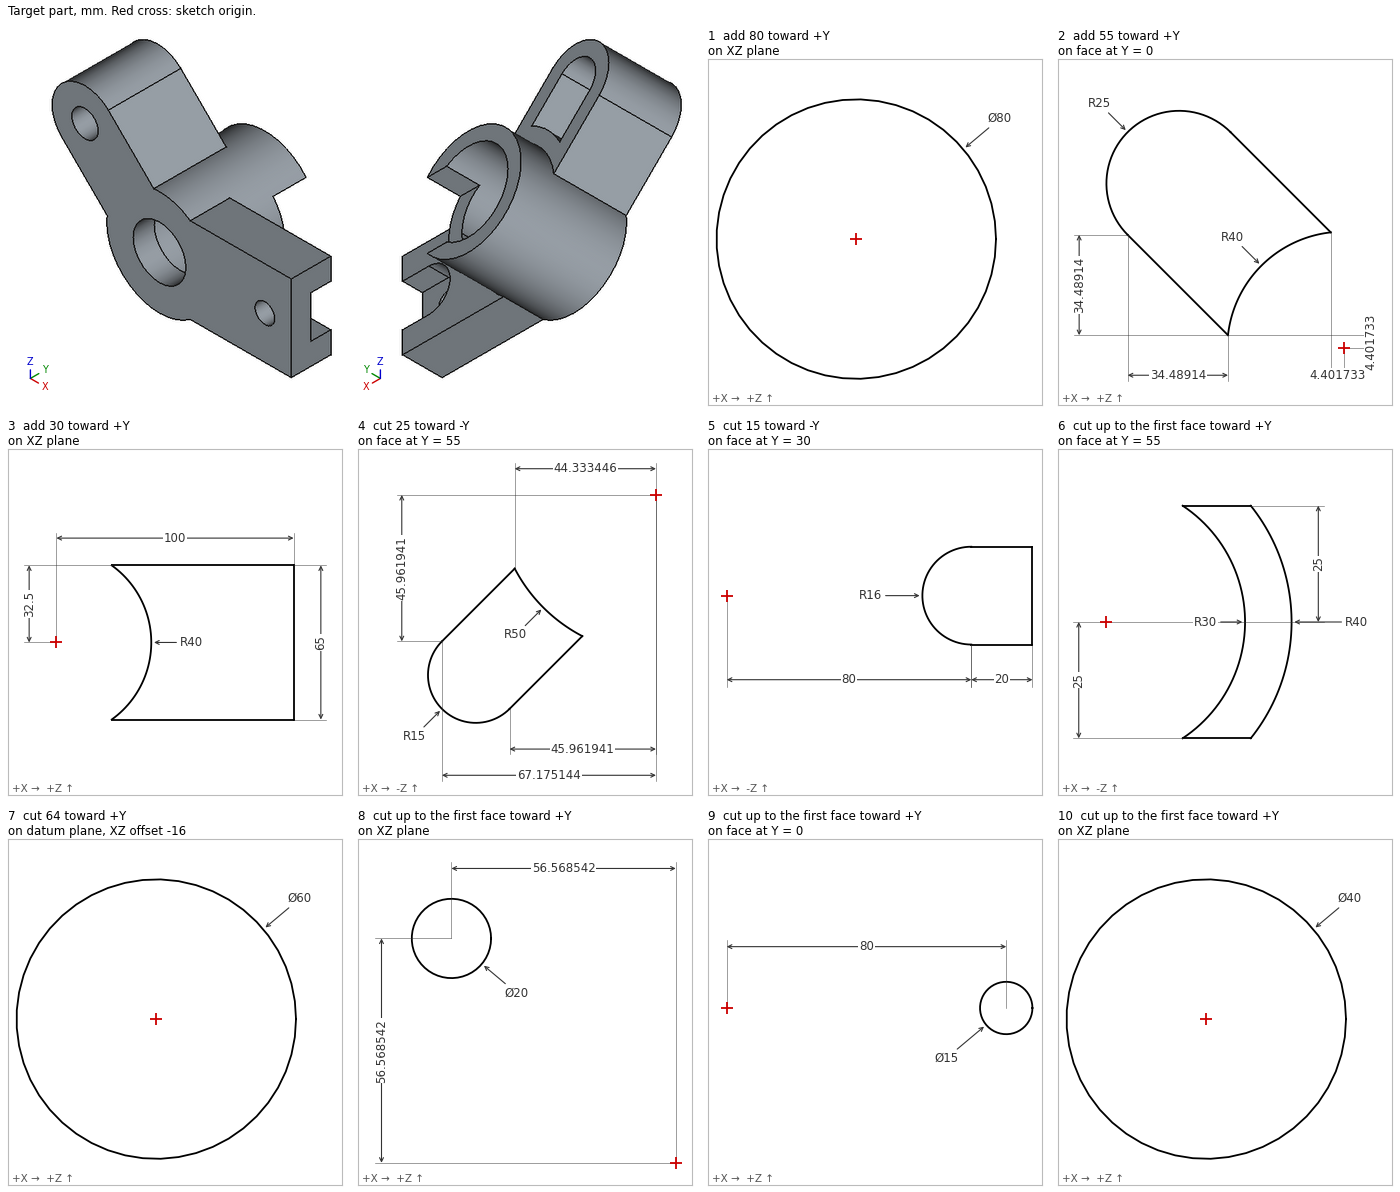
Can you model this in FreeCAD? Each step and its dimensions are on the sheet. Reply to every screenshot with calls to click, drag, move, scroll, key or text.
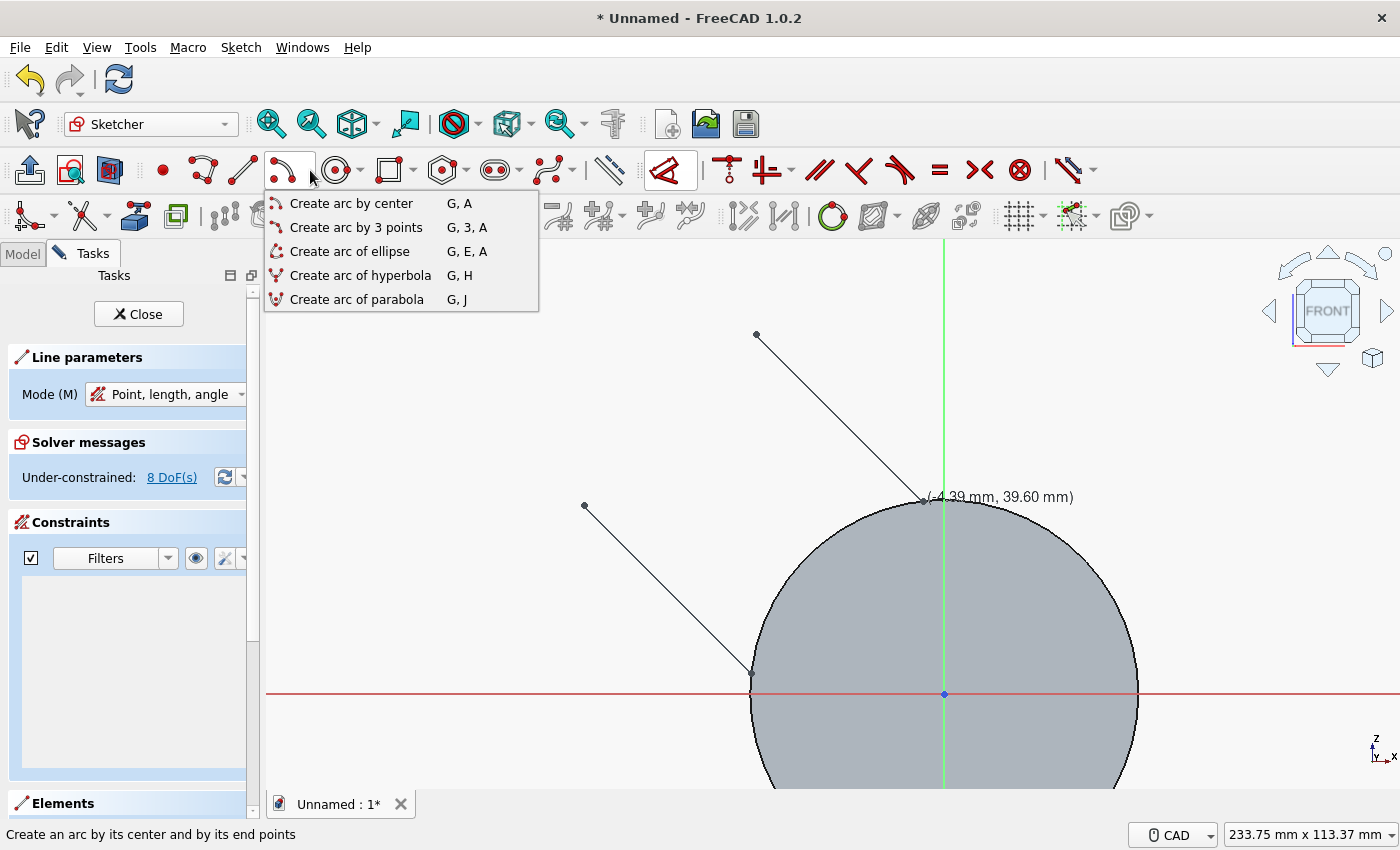
click(402, 227)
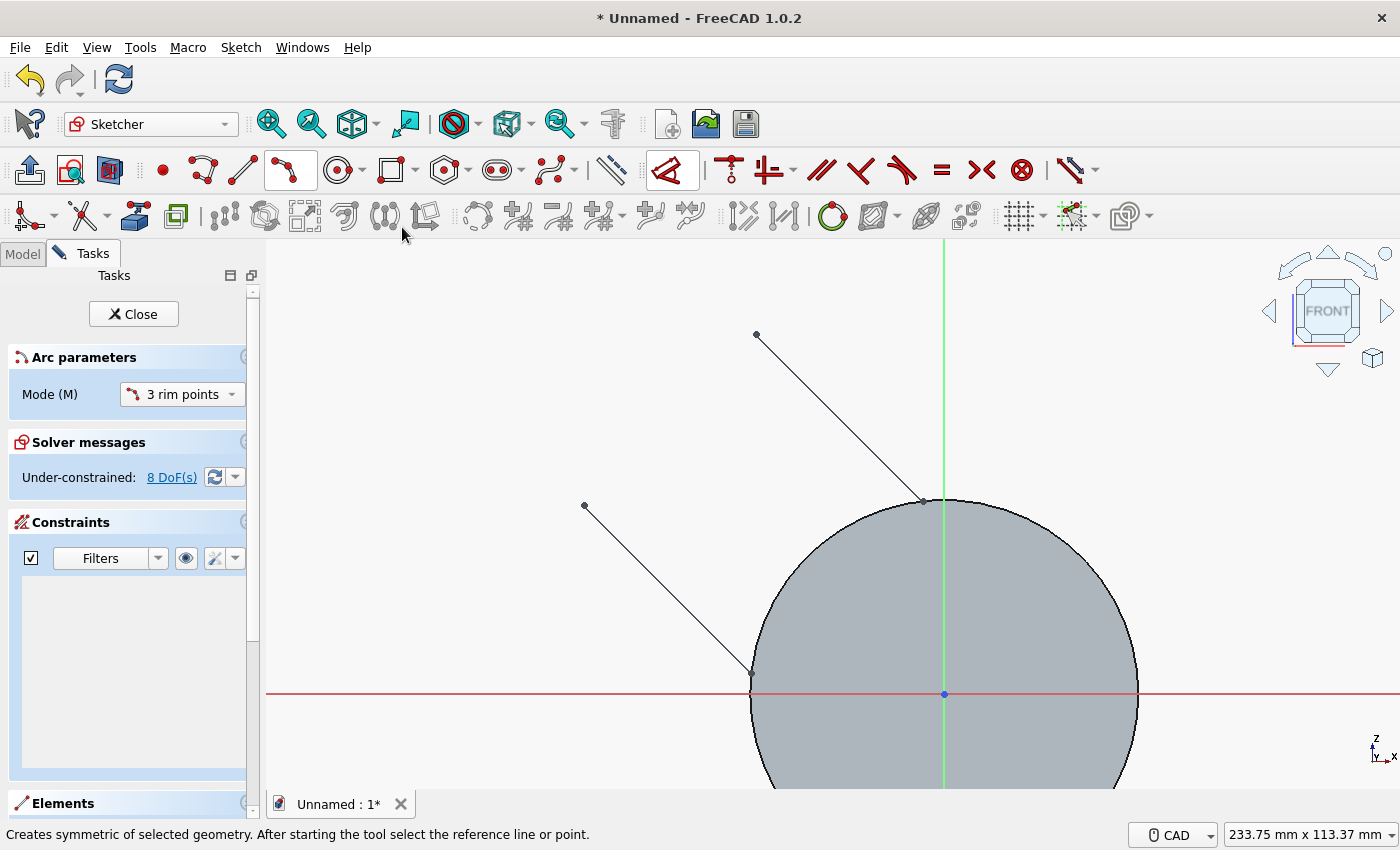
click(584, 506)
click(756, 335)
click(584, 334)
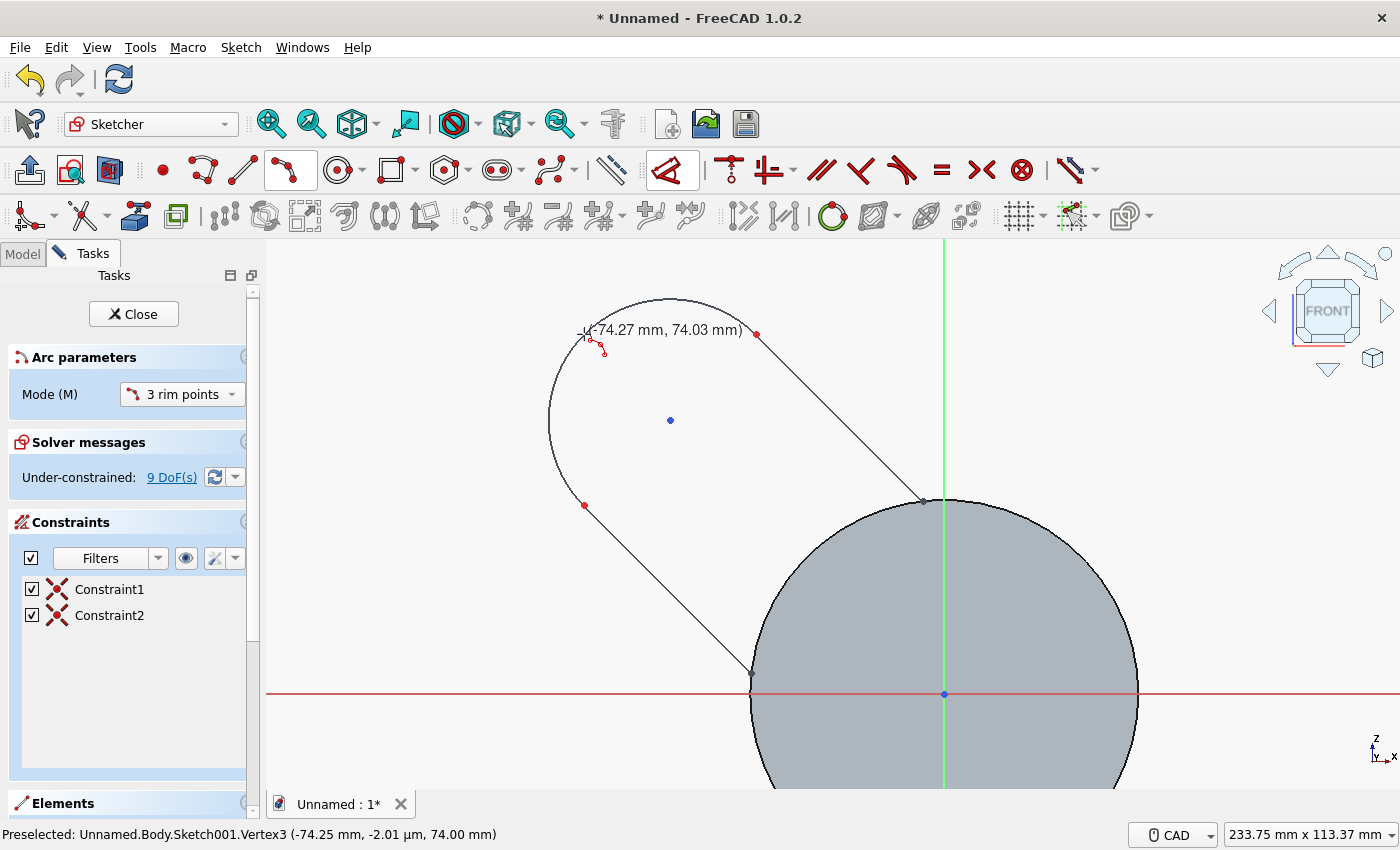
click(923, 502)
click(751, 674)
click(807, 557)
key(Escape)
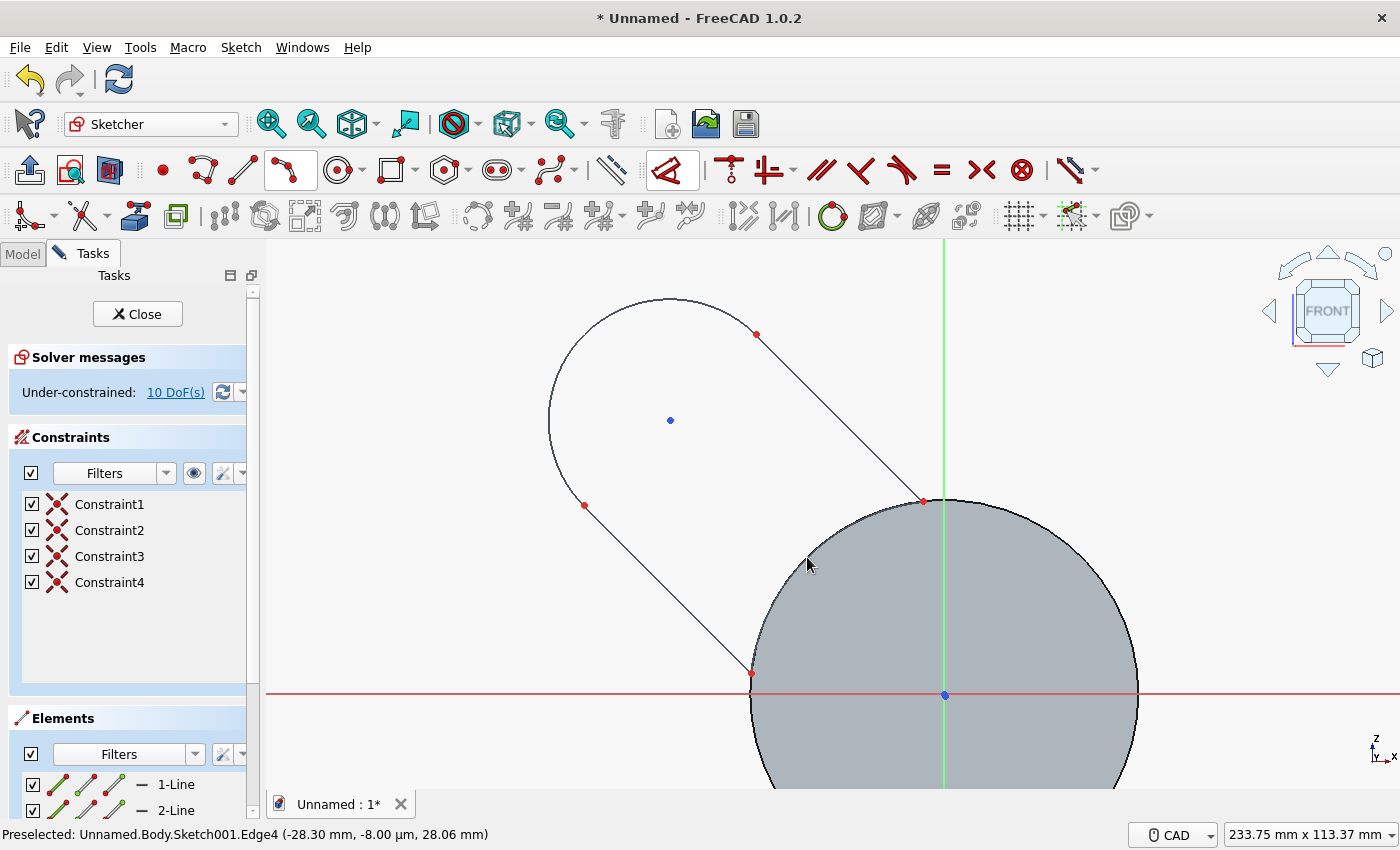
click(701, 624)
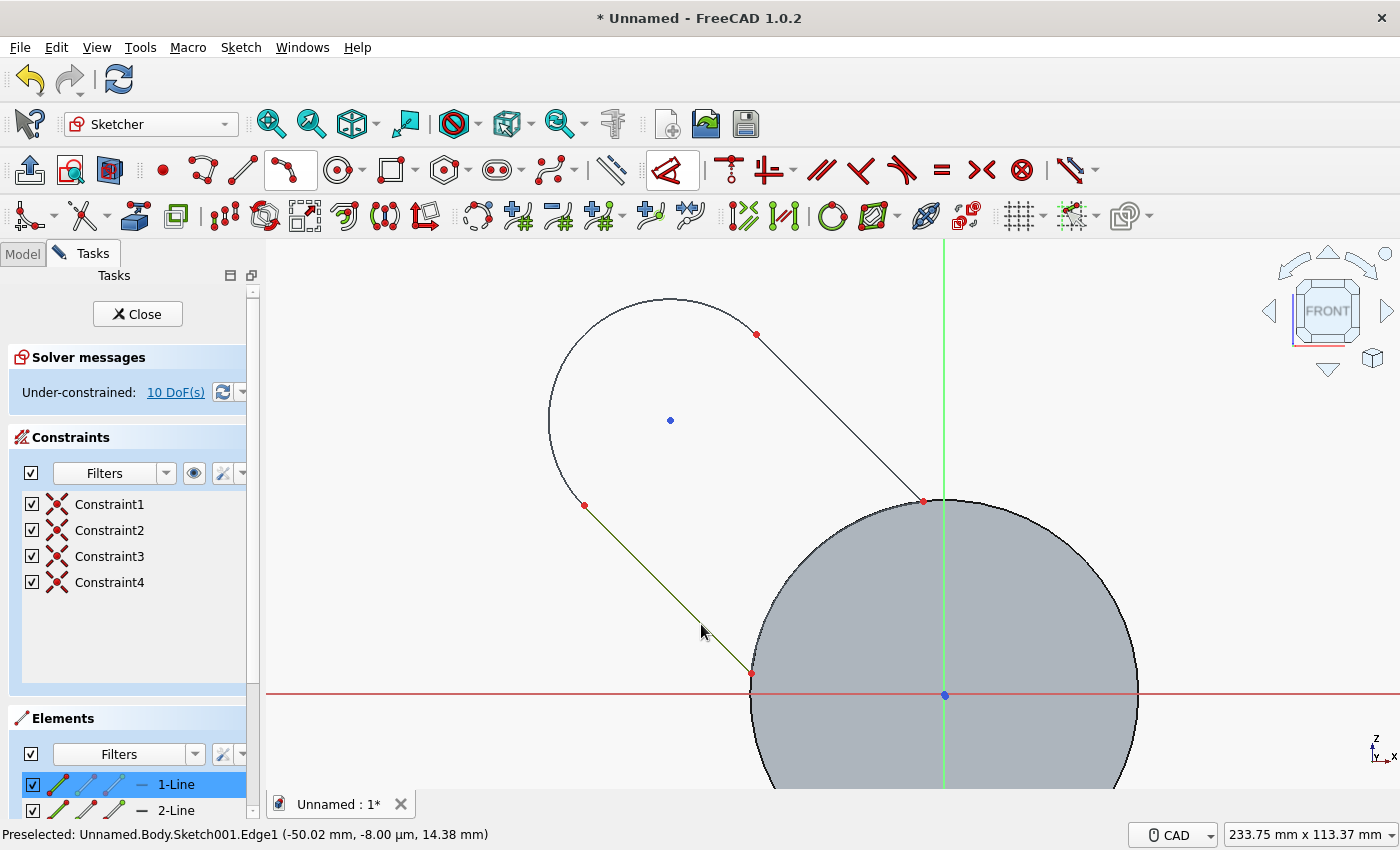
click(651, 301)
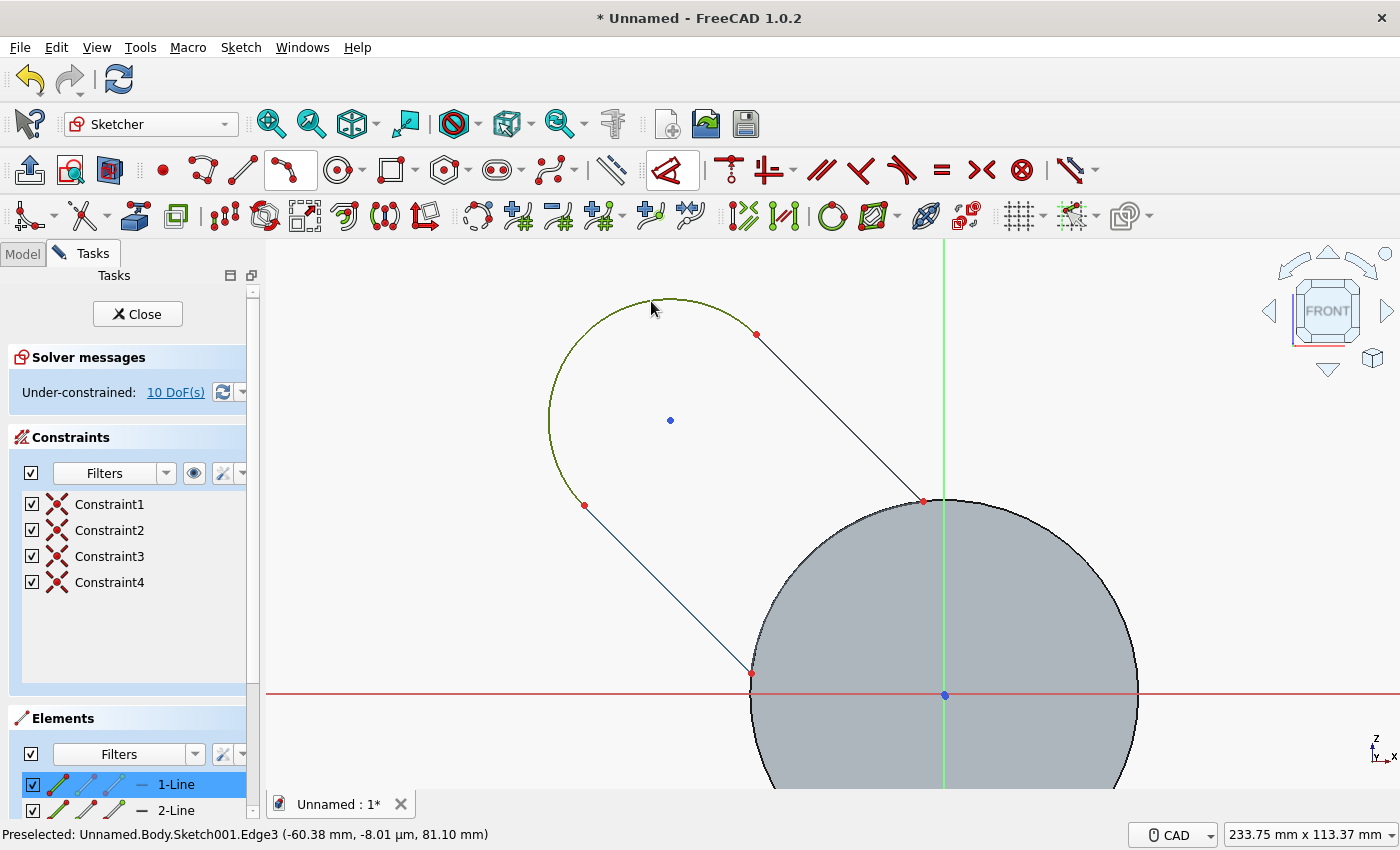
click(902, 170)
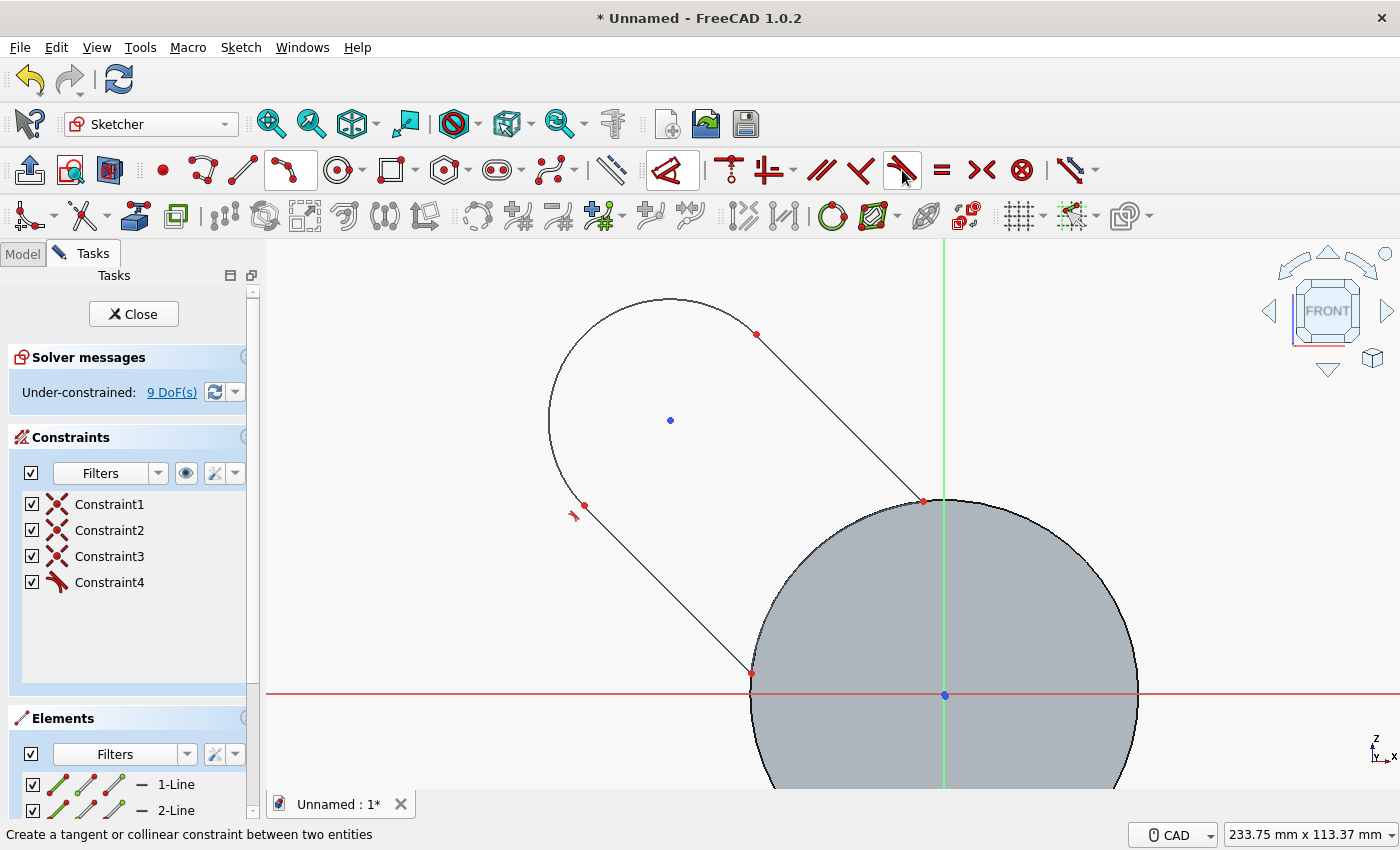
click(806, 385)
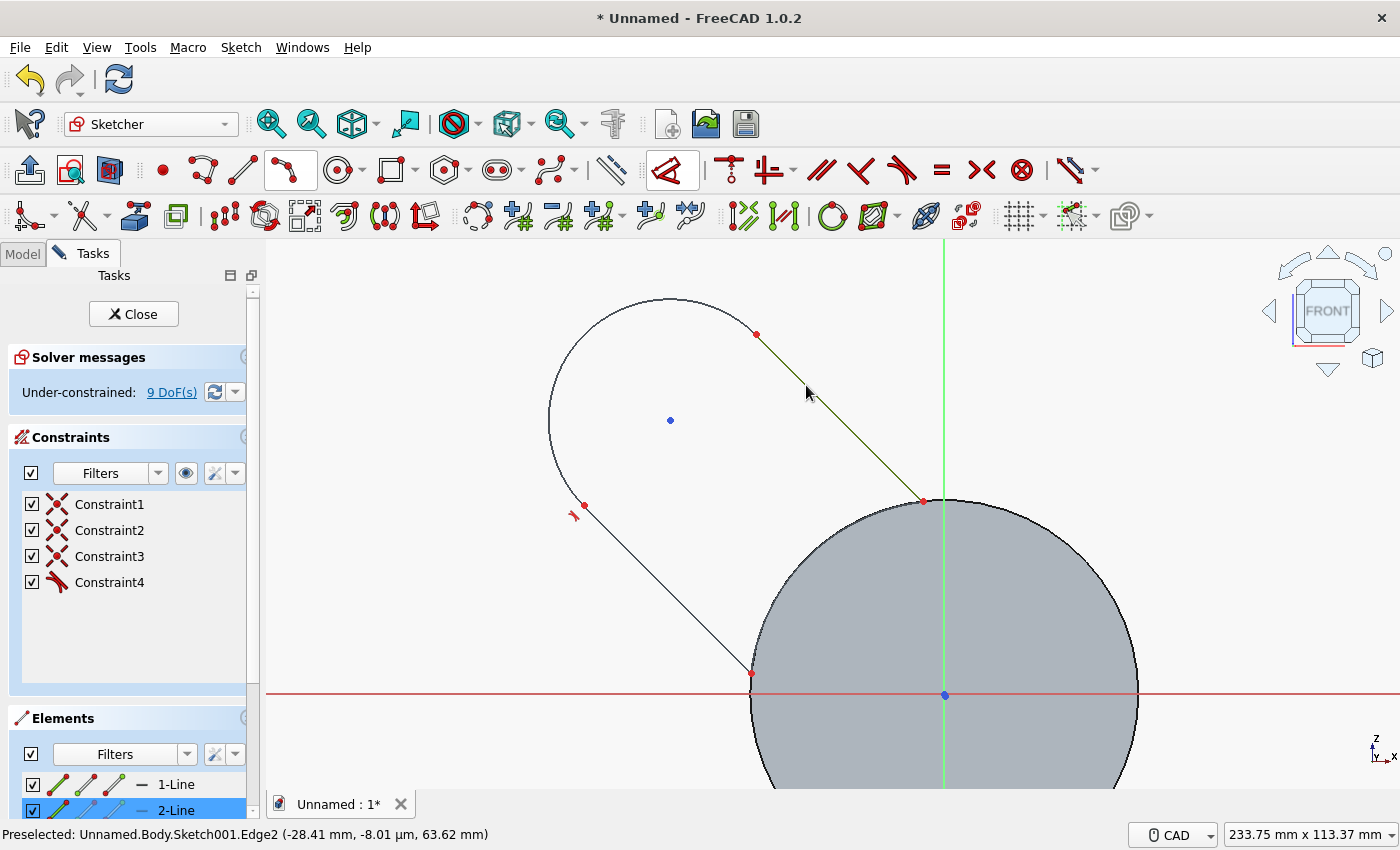
click(651, 301)